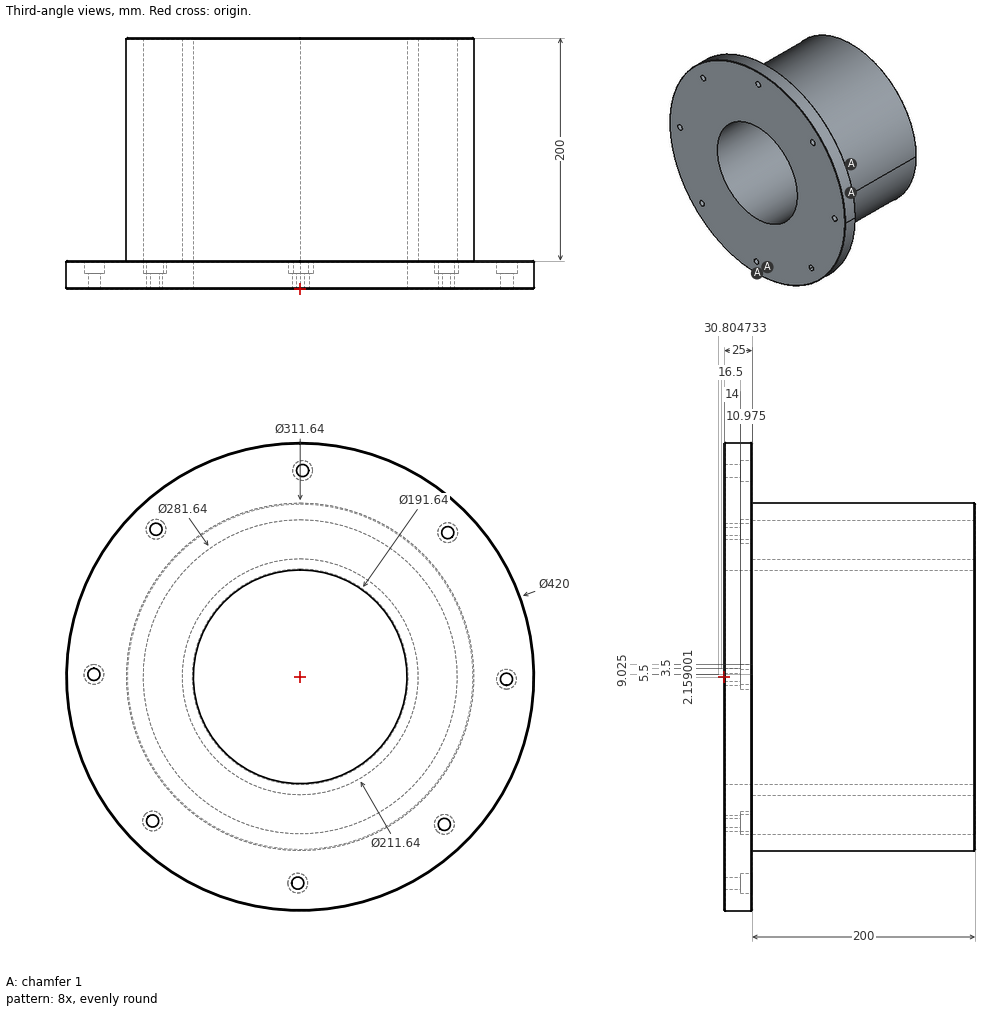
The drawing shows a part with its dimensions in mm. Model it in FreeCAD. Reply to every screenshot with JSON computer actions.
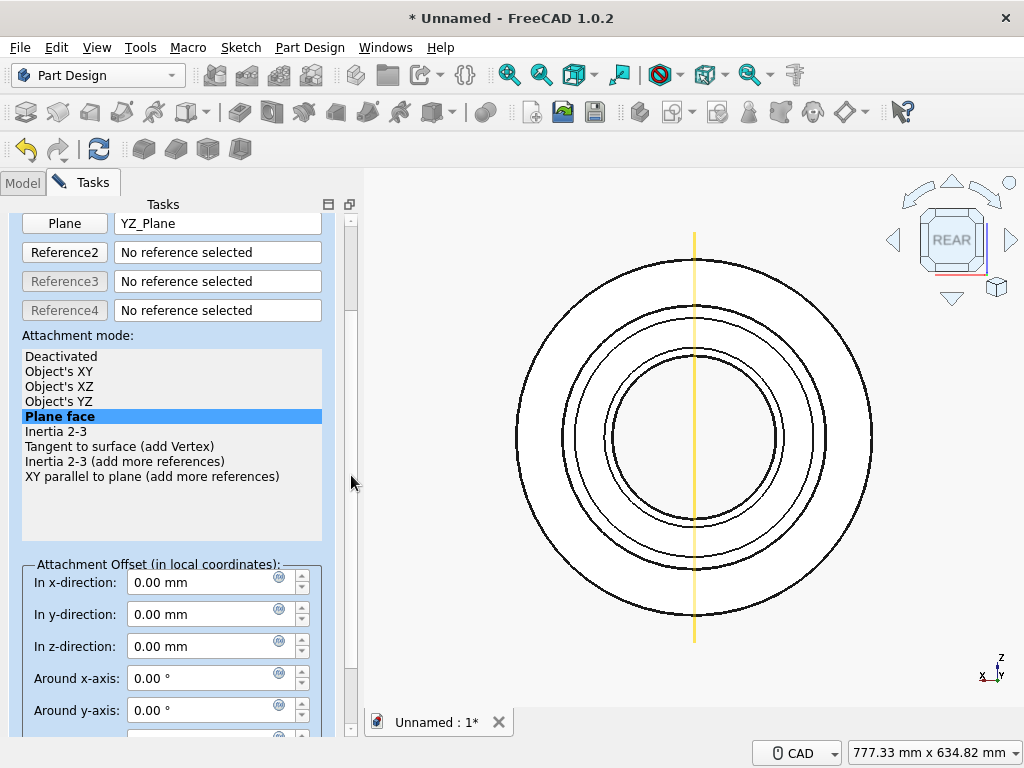
{"action": "triple_click", "coordinate": [210, 646]}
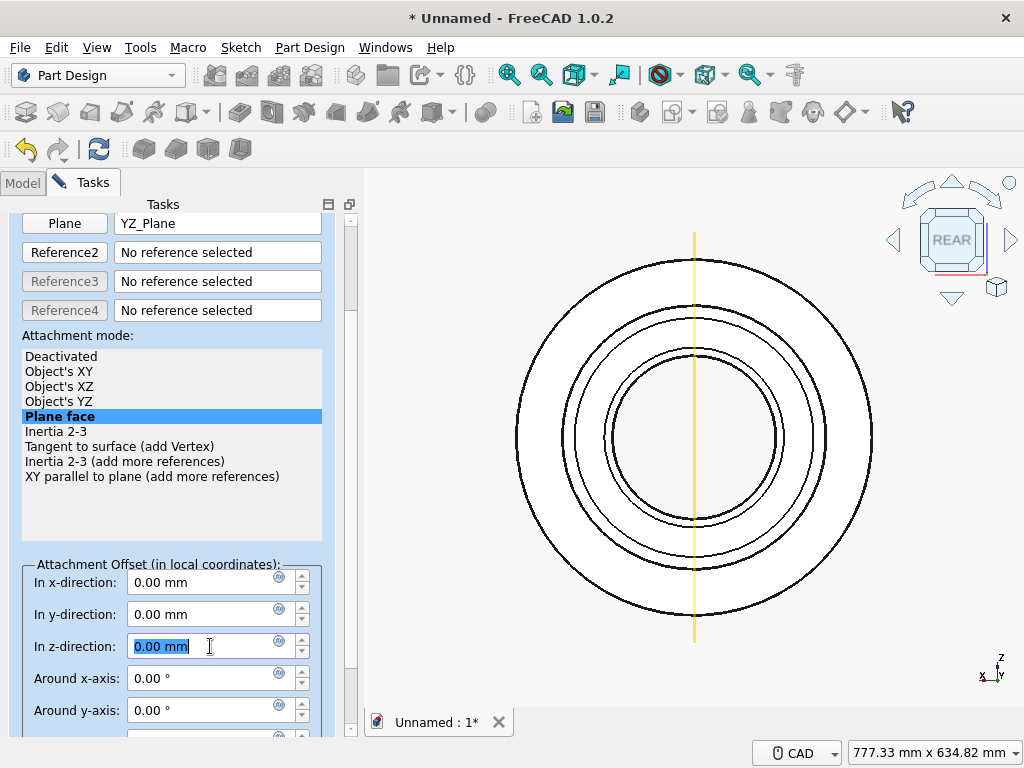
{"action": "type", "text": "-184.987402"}
{"action": "key", "text": "Tab"}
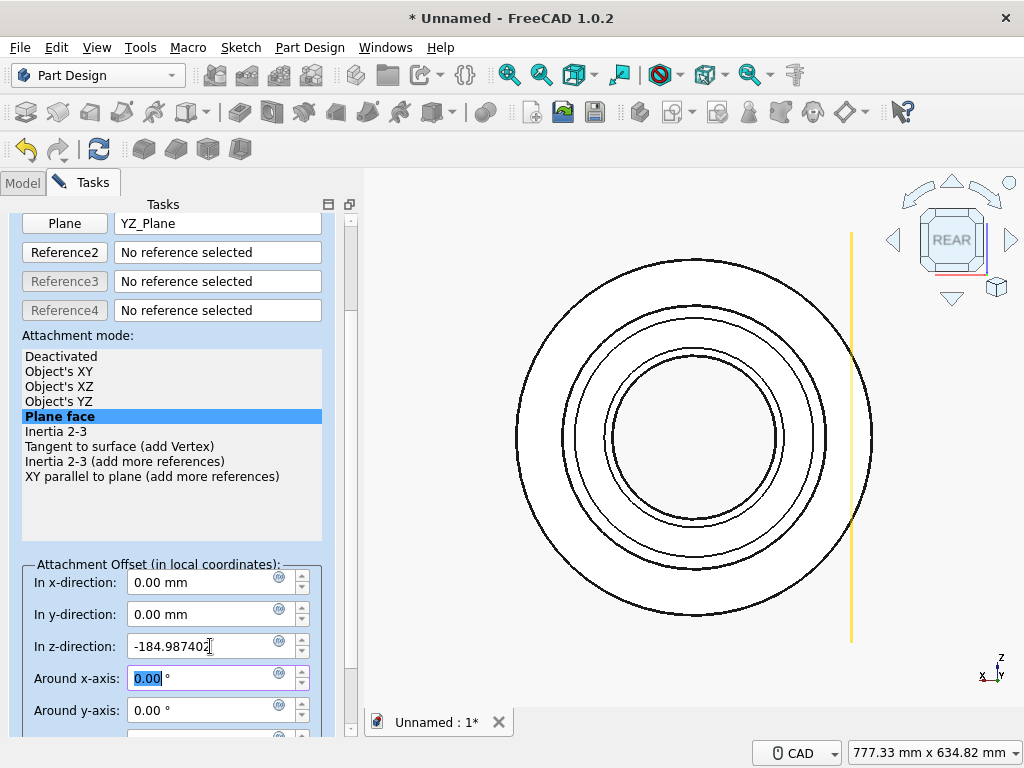
{"action": "scroll", "coordinate": [351, 475], "scroll_direction": "up", "scroll_amount": 3}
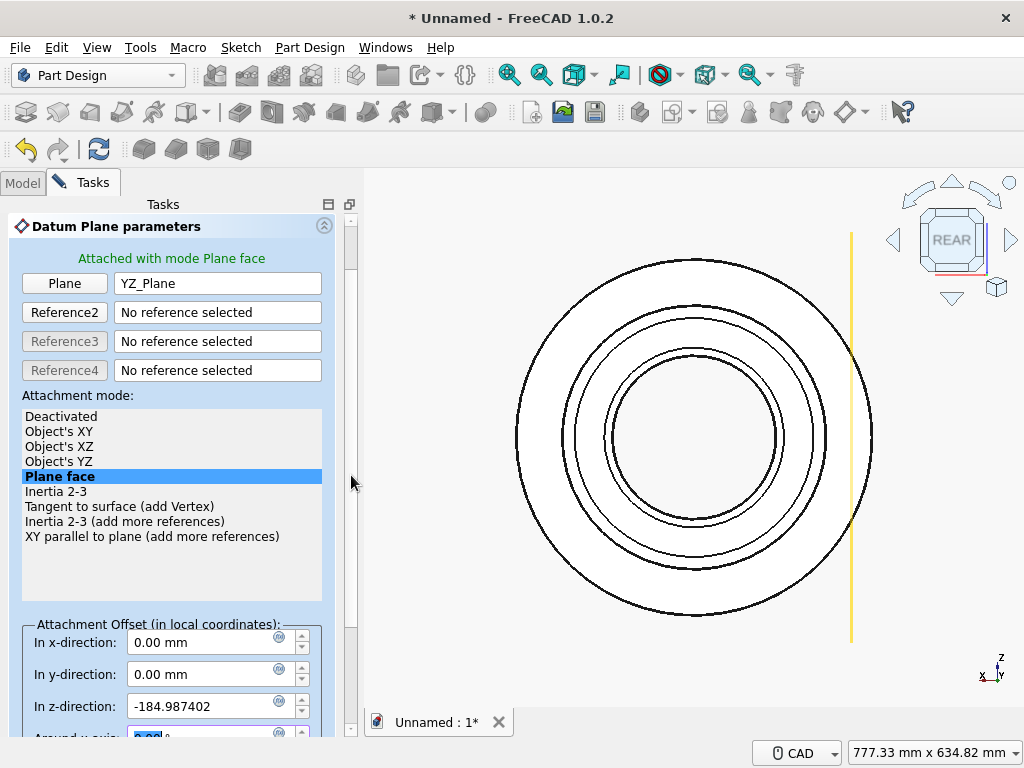
{"action": "left_click", "coordinate": [124, 243]}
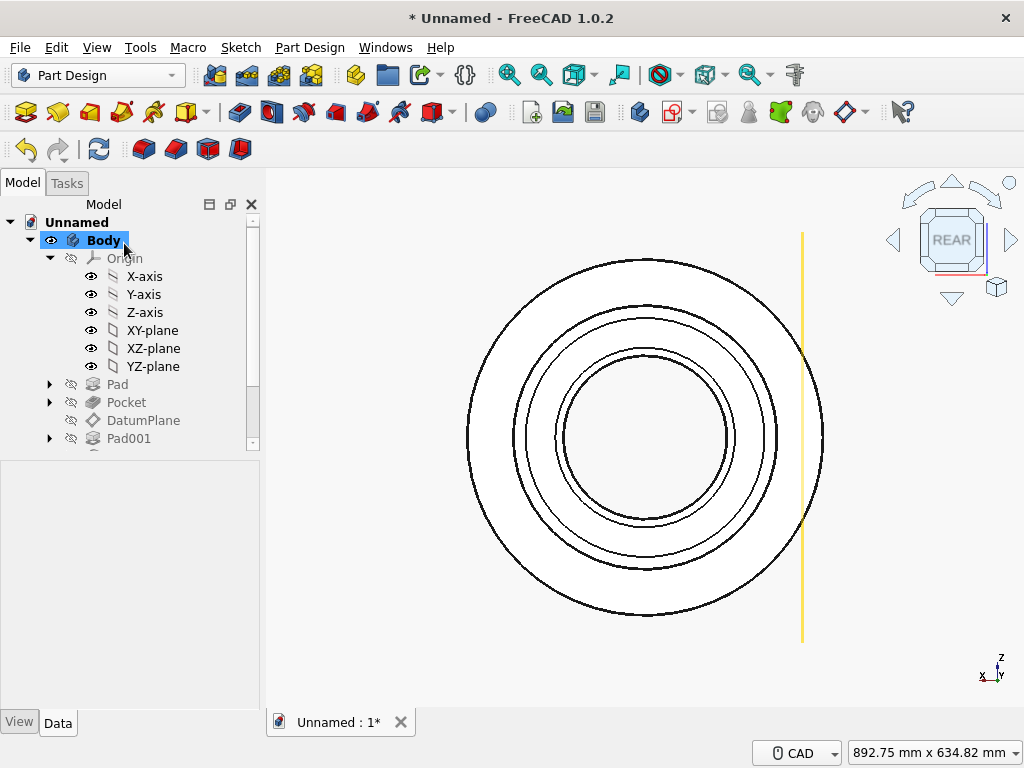
{"action": "scroll", "coordinate": [100, 326], "scroll_direction": "down", "scroll_amount": 3}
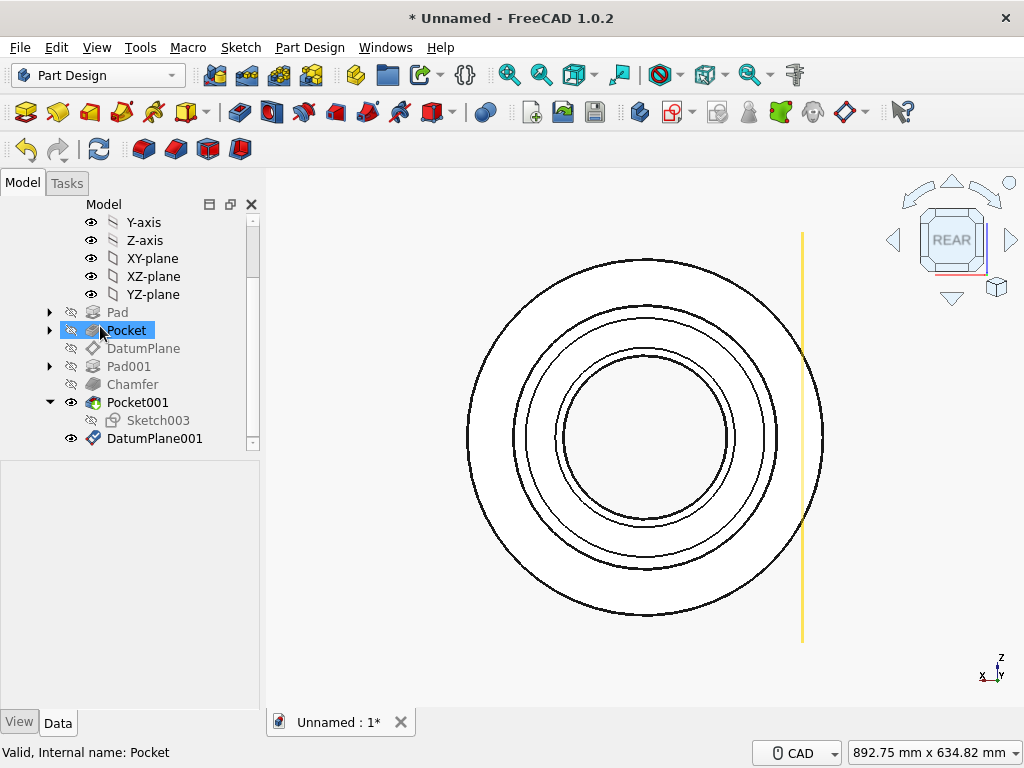
{"action": "left_click", "coordinate": [116, 438]}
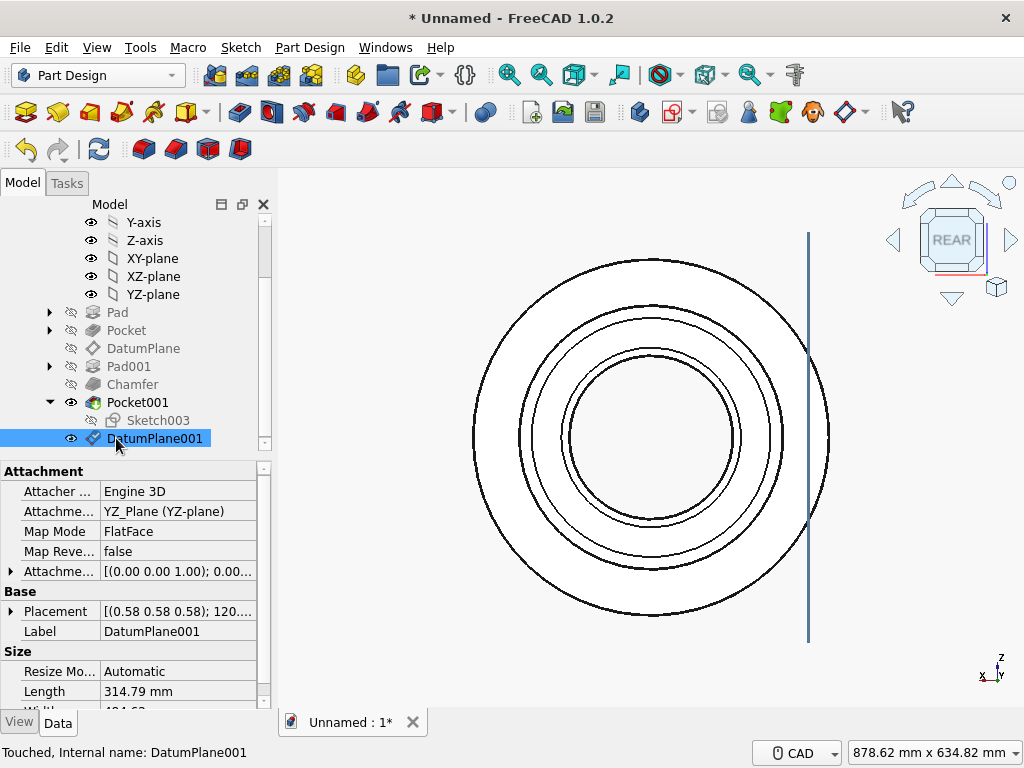
{"action": "left_click", "coordinate": [672, 112]}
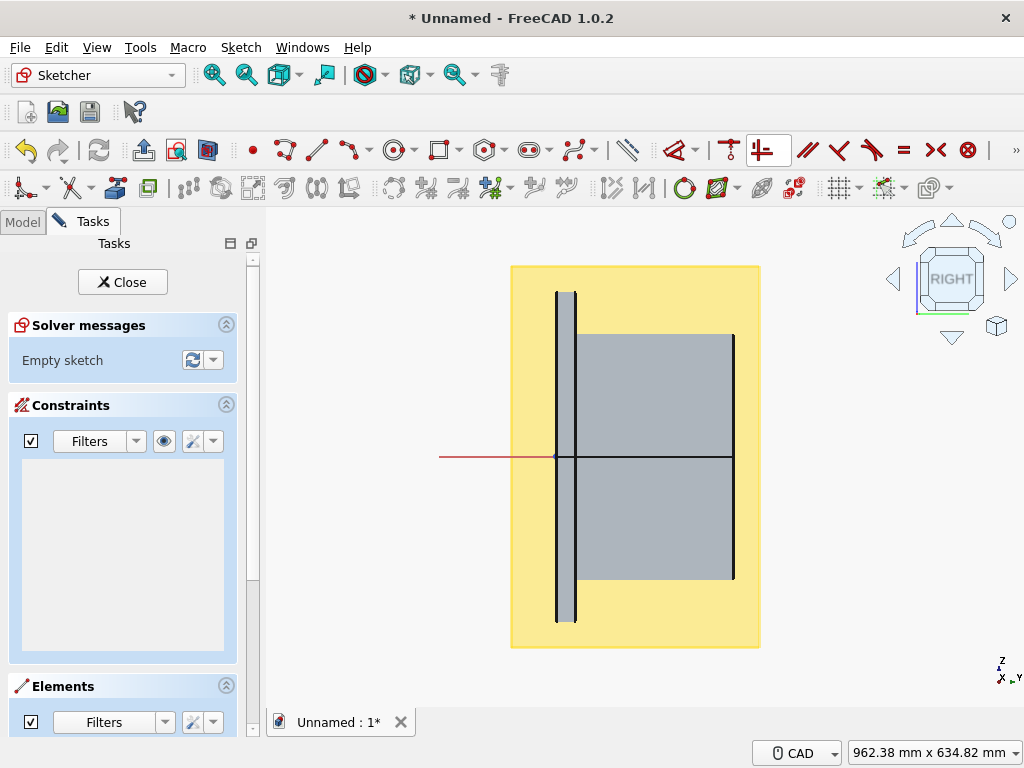
{"action": "left_click", "coordinate": [208, 150]}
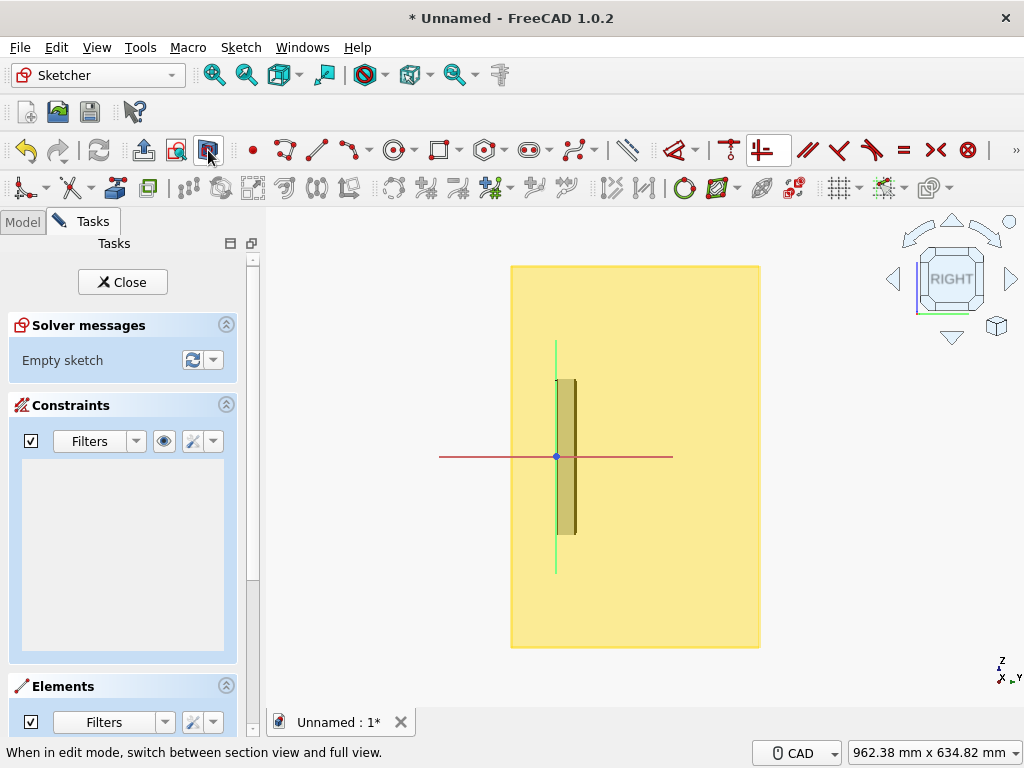
{"action": "scroll", "coordinate": [557, 452], "scroll_direction": "up", "scroll_amount": 12}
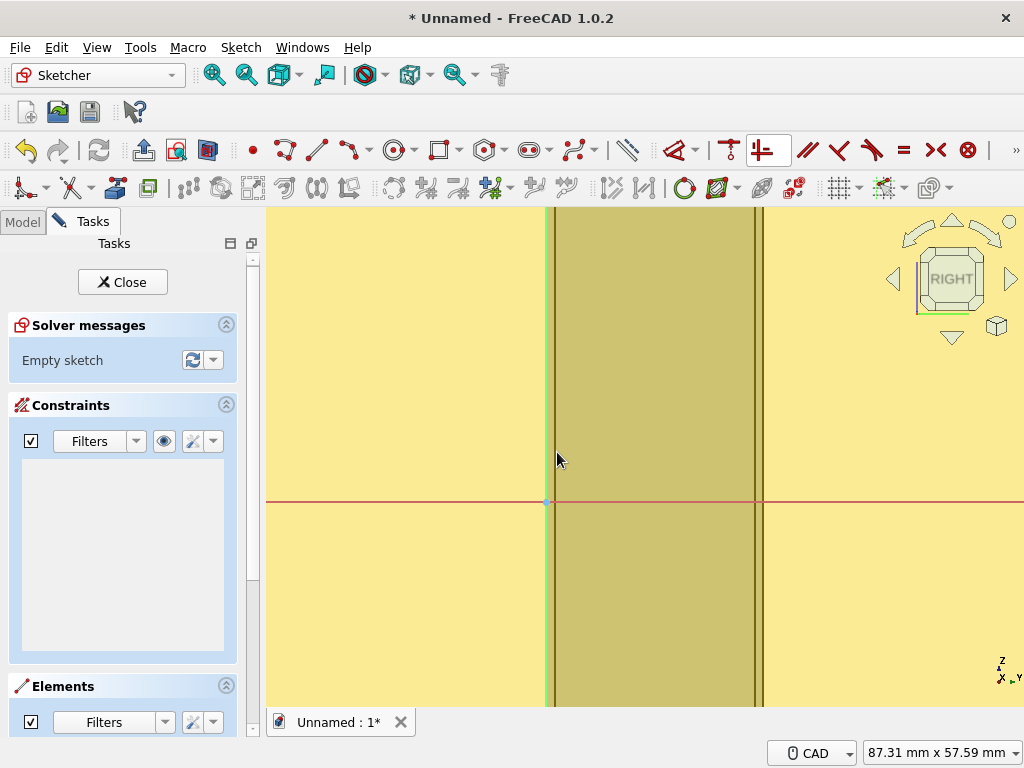
{"action": "left_click", "coordinate": [286, 150]}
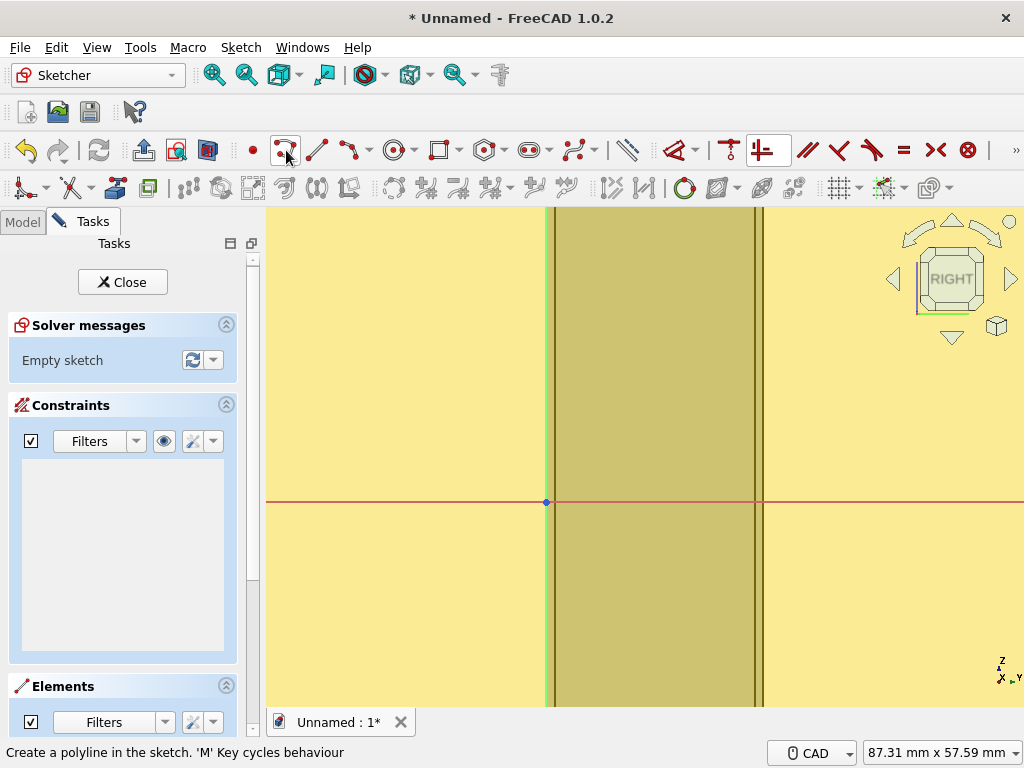
{"action": "left_click", "coordinate": [496, 483]}
{"action": "left_click", "coordinate": [763, 483]}
{"action": "left_click", "coordinate": [763, 405]}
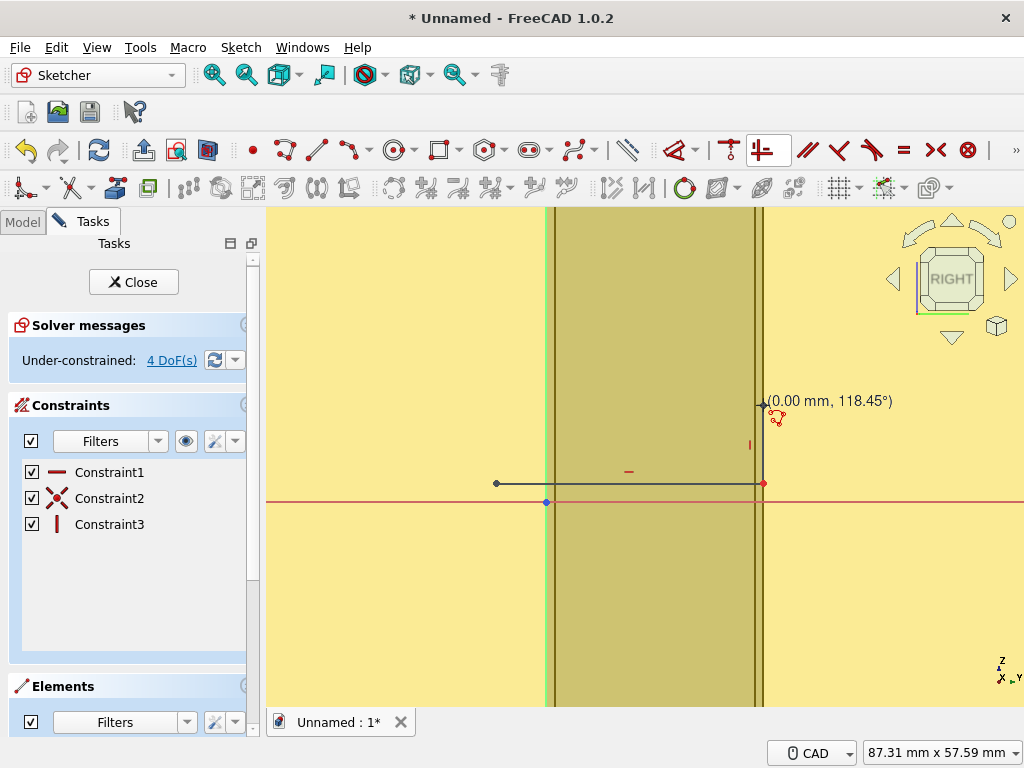
{"action": "scroll", "coordinate": [763, 405], "scroll_direction": "up", "scroll_amount": 22}